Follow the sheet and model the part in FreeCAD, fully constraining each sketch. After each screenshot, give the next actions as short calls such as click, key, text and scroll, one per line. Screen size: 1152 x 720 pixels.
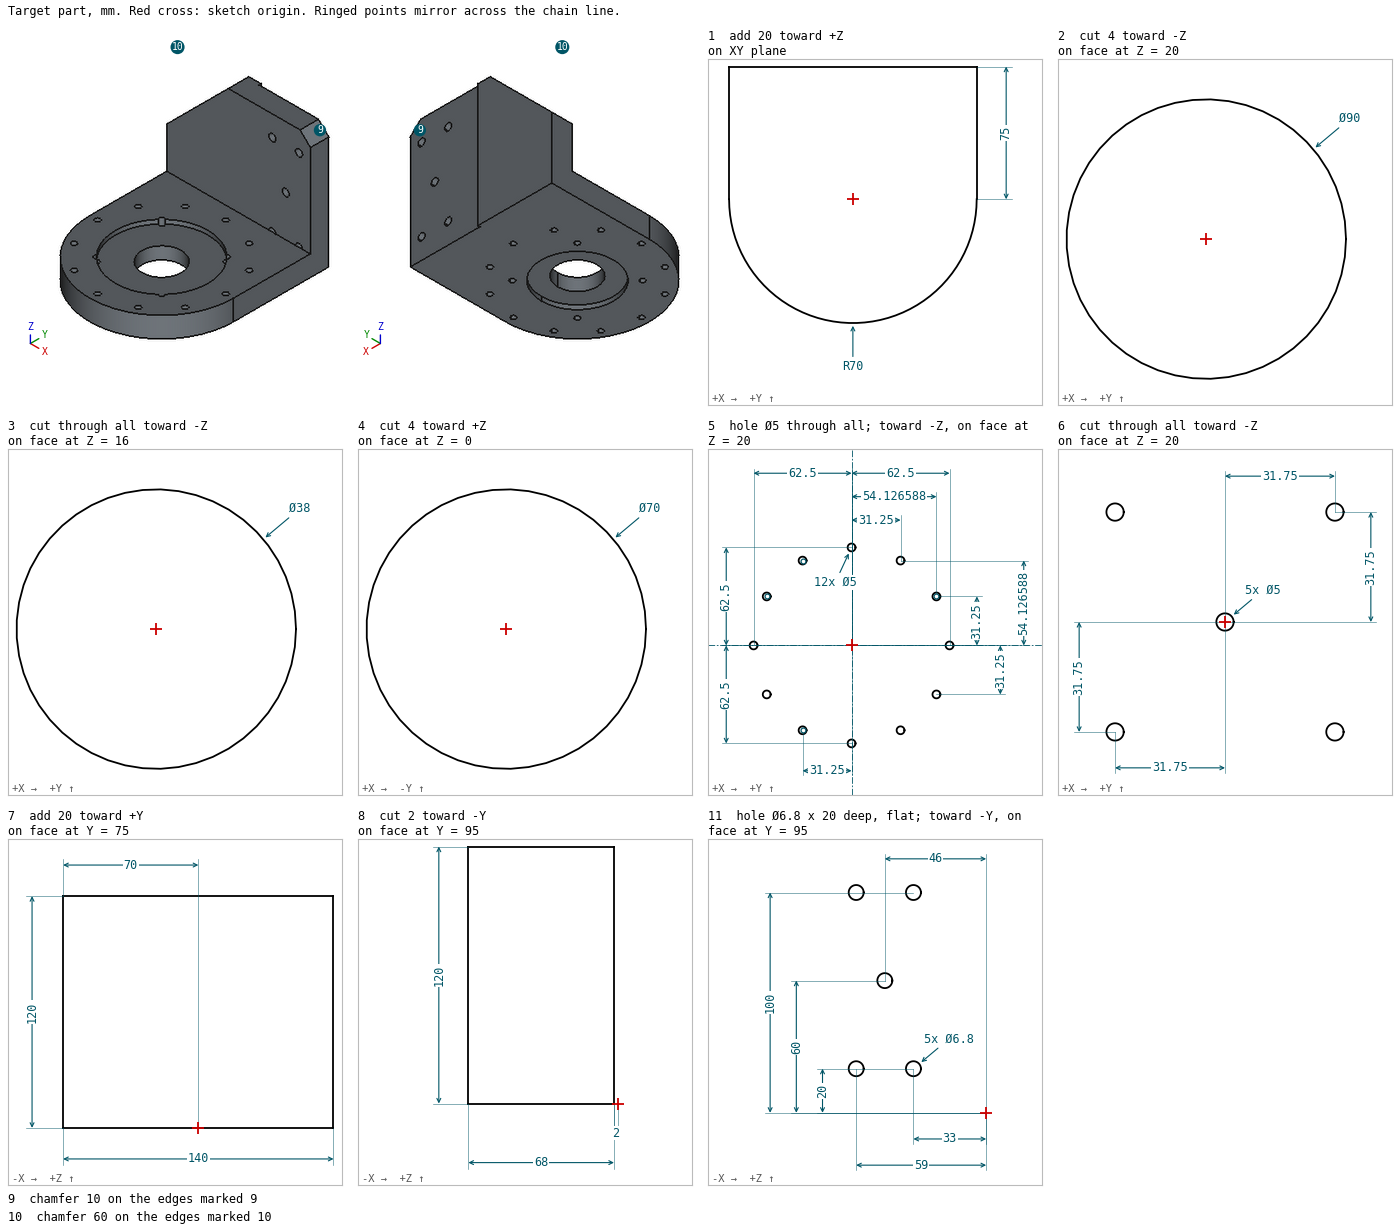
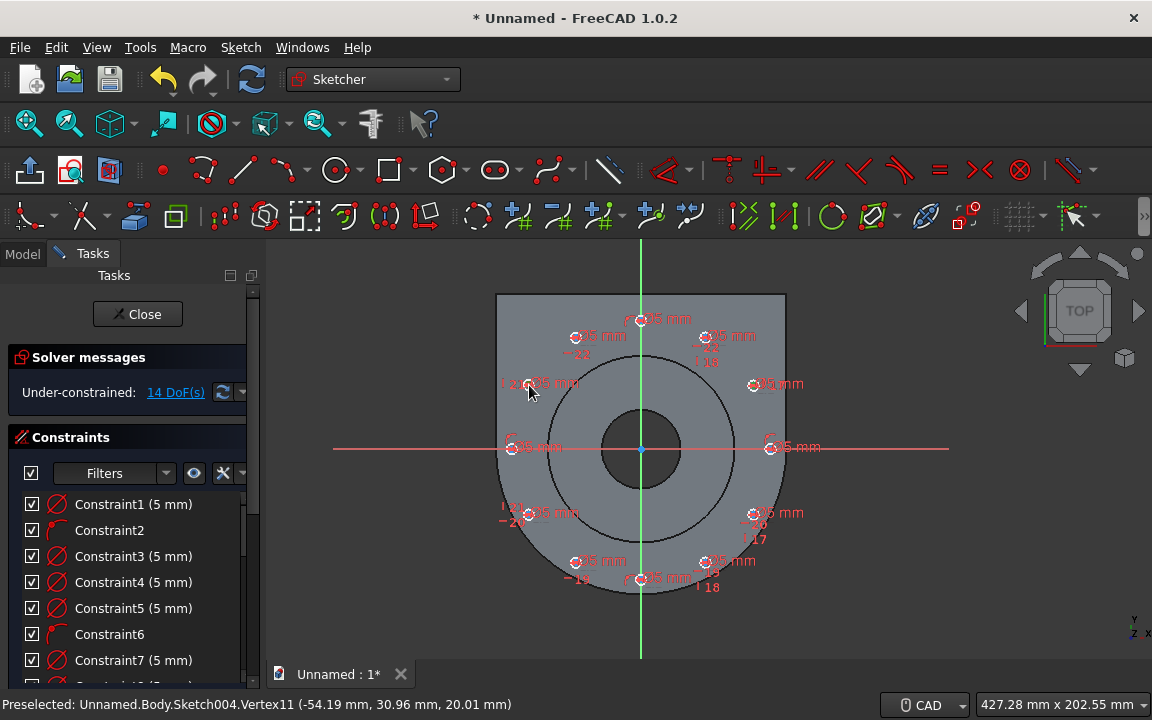
click(641, 527)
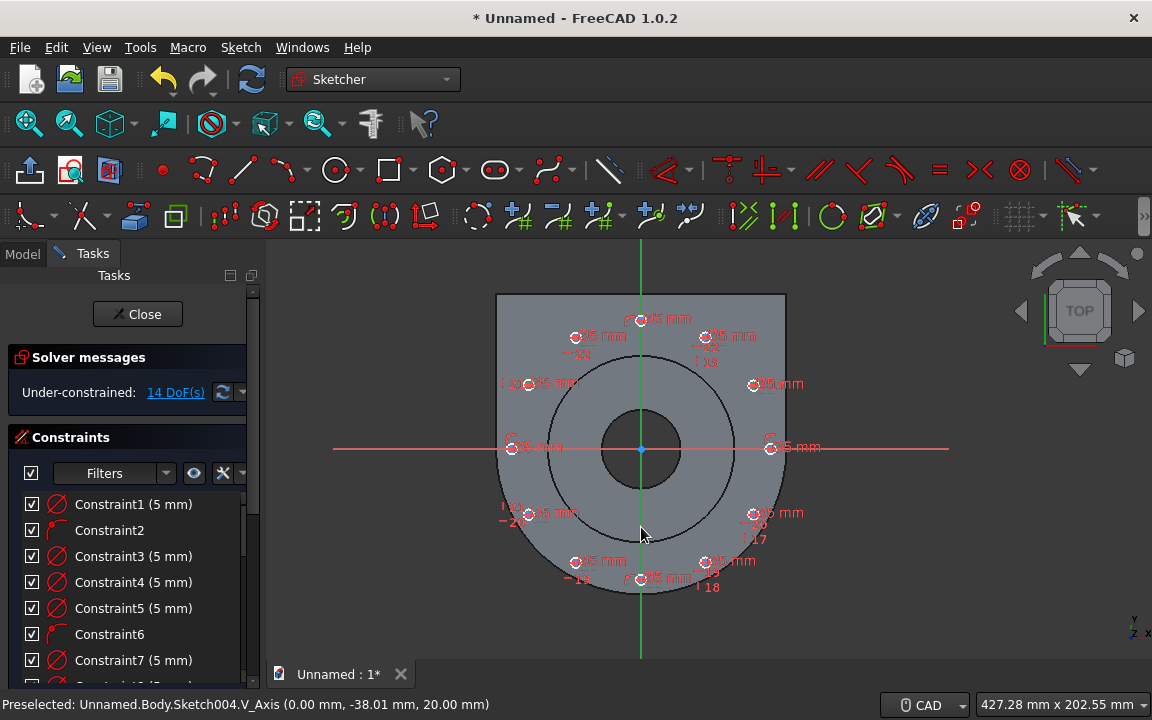
click(980, 170)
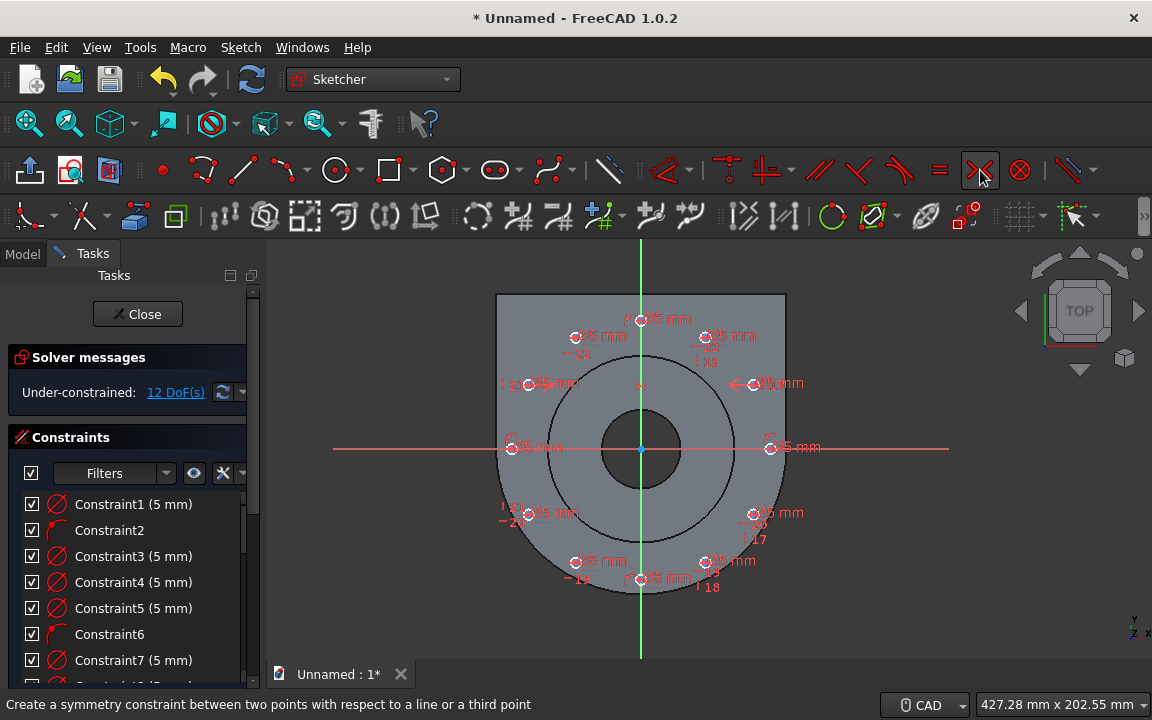
click(576, 563)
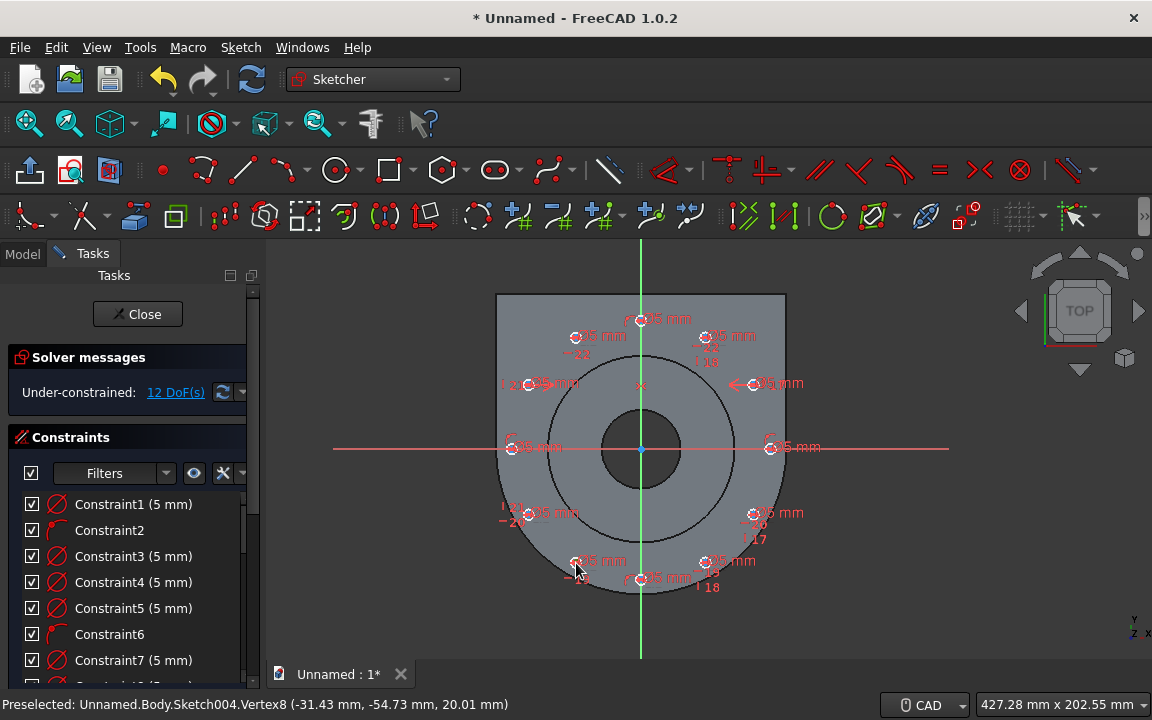
click(576, 338)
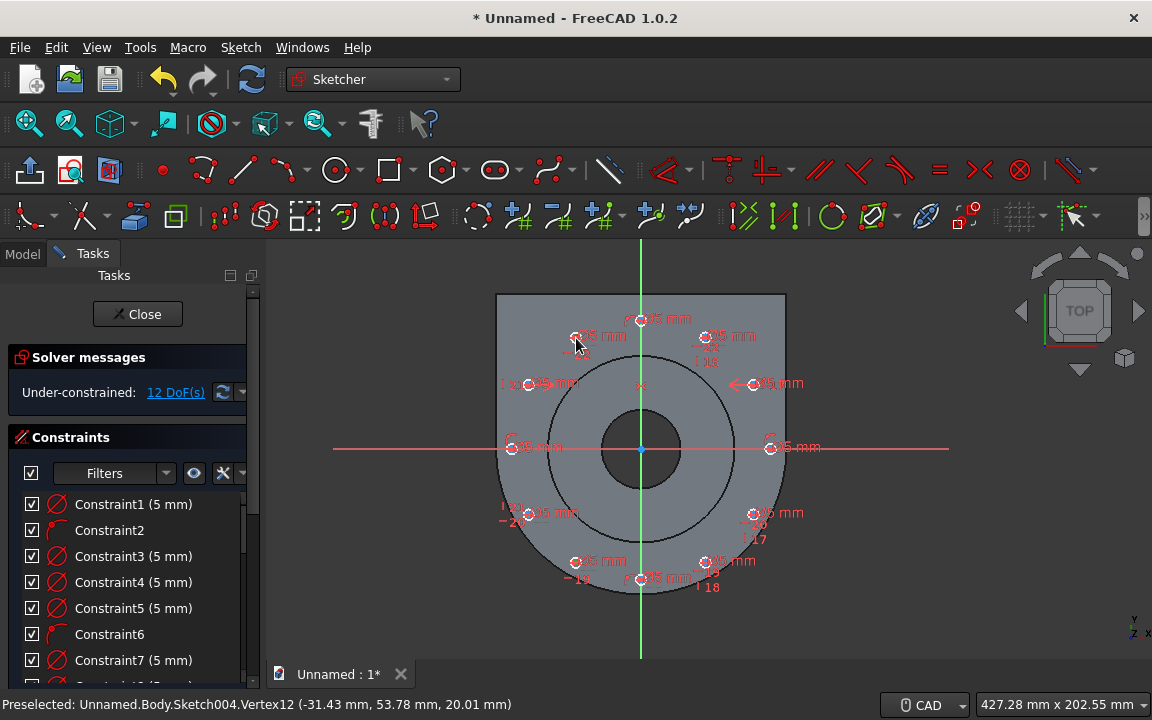
click(343, 449)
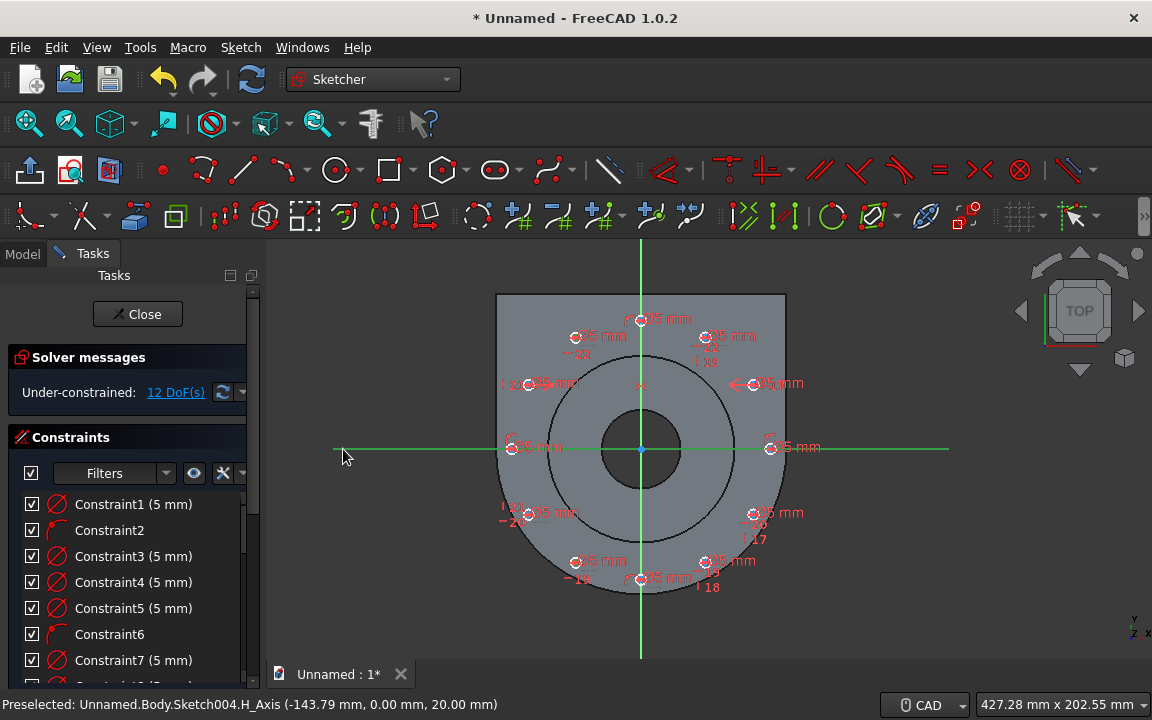
key(s)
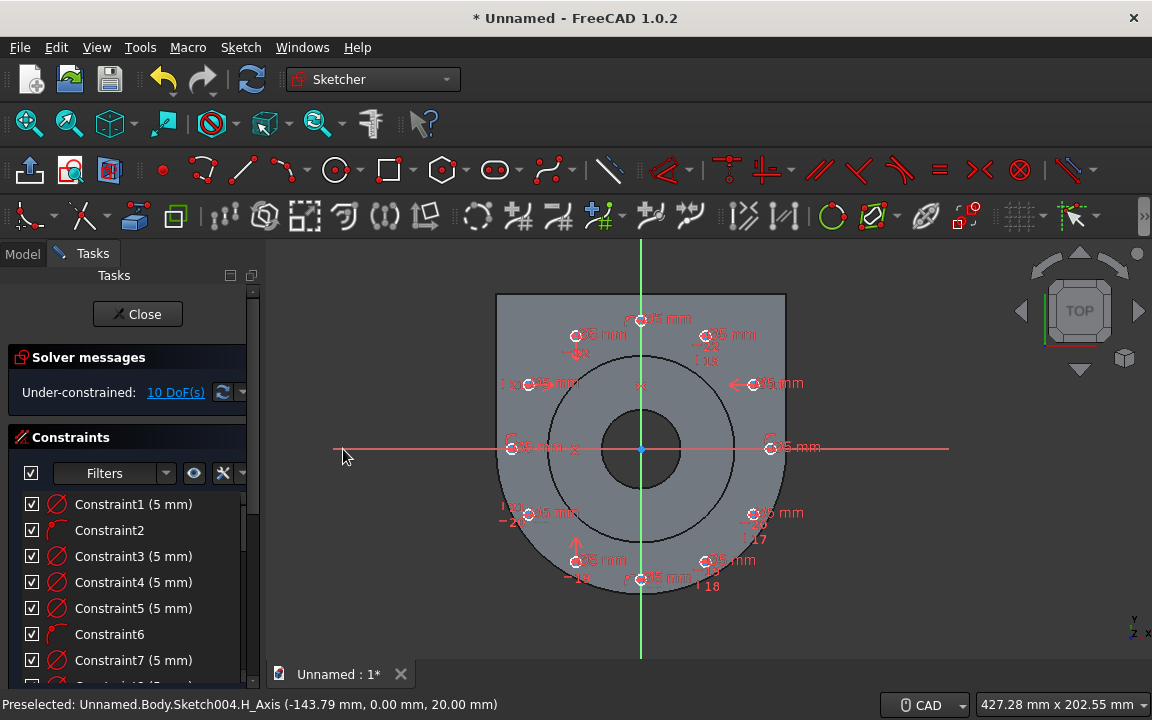
click(664, 170)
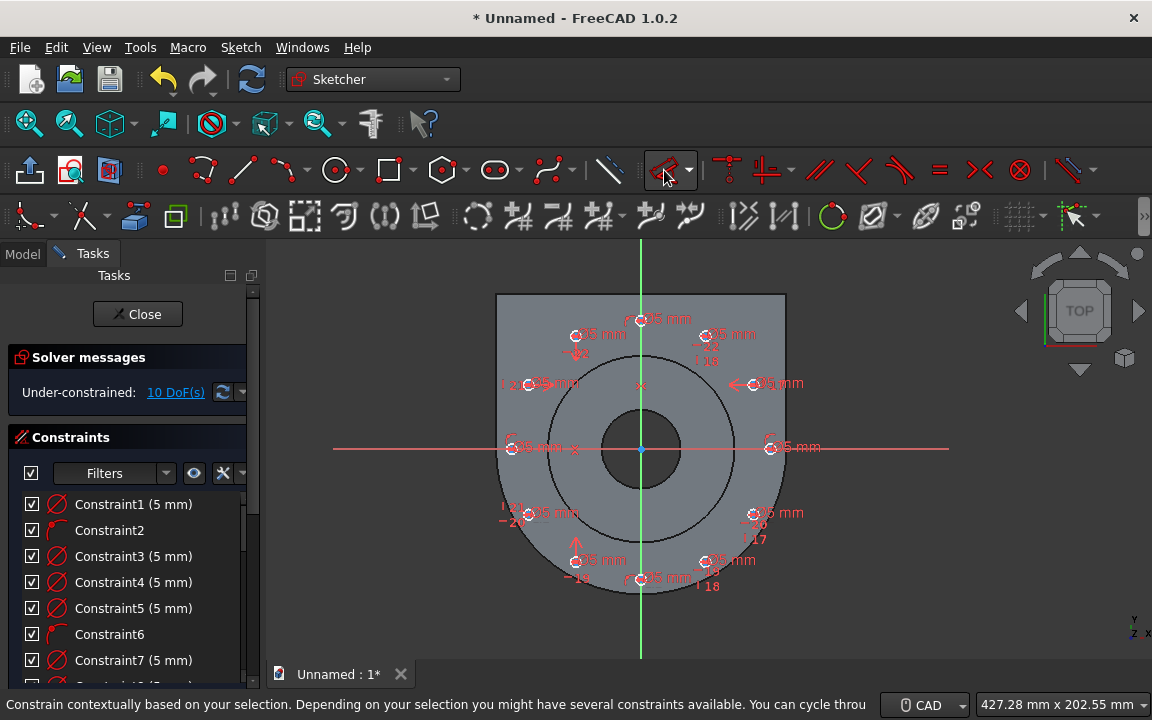
click(641, 321)
click(675, 385)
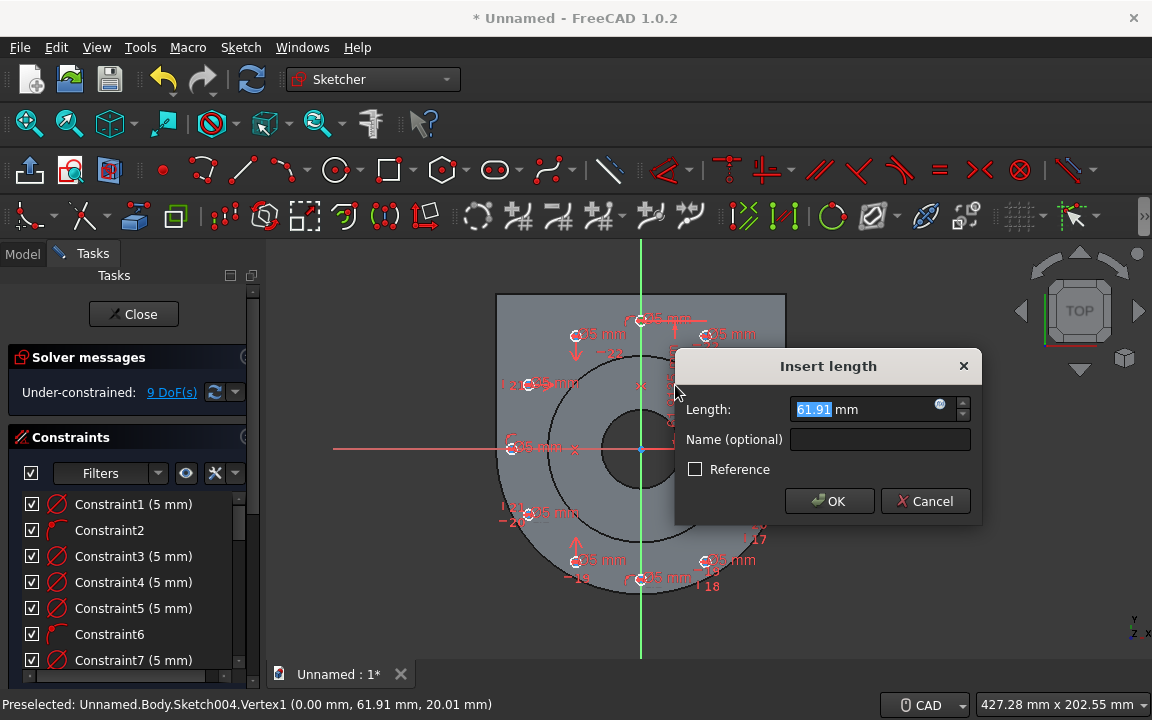
text(62.5)
key(Return)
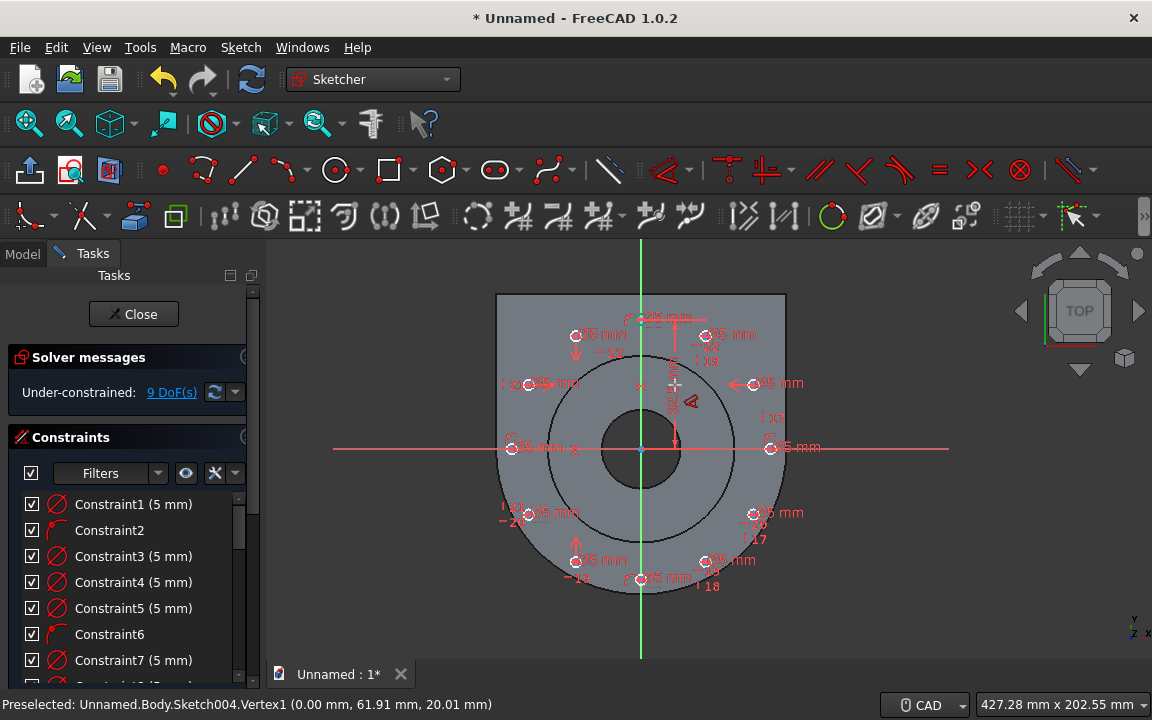
click(771, 449)
click(706, 483)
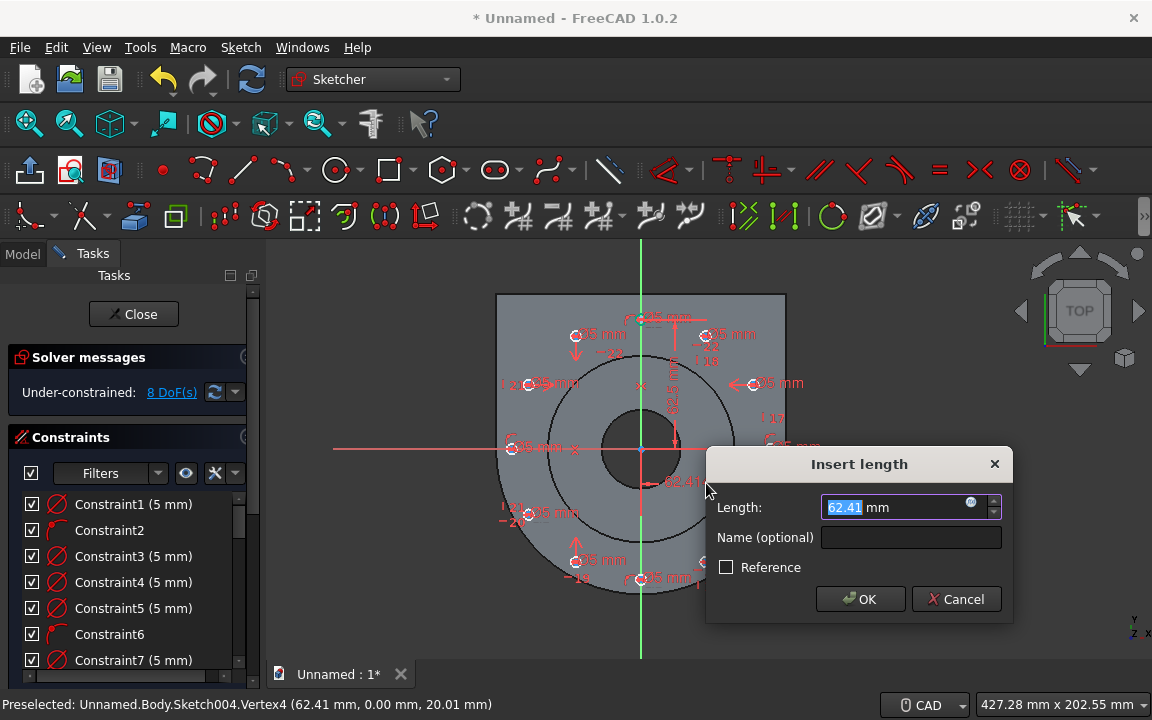
text(62.5)
key(Return)